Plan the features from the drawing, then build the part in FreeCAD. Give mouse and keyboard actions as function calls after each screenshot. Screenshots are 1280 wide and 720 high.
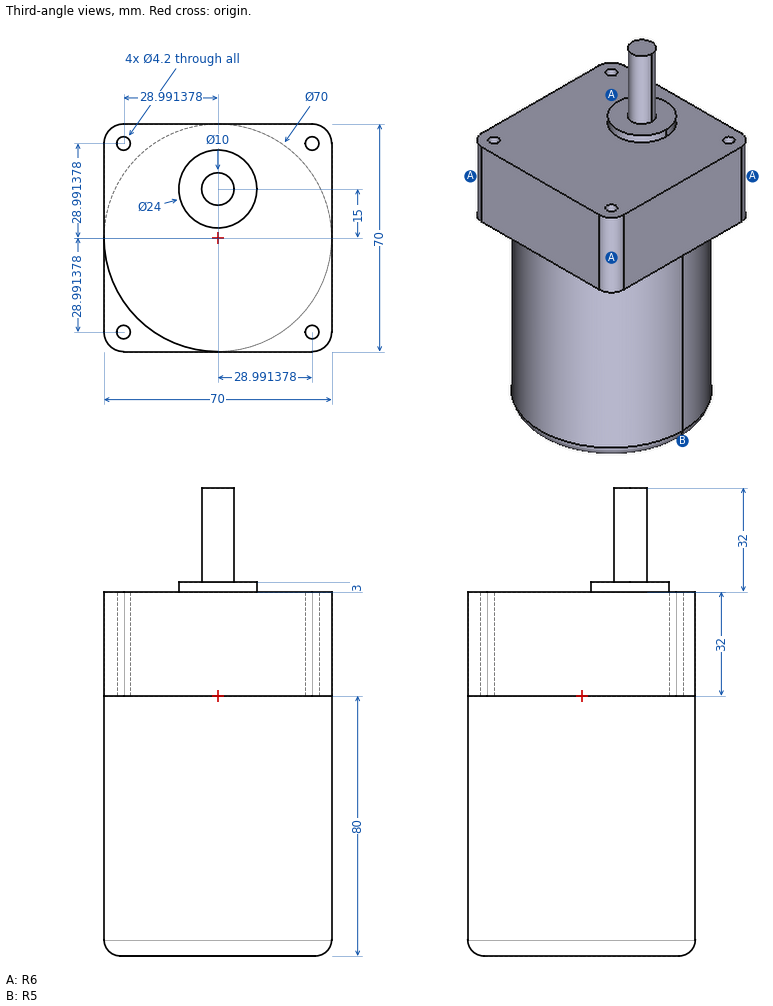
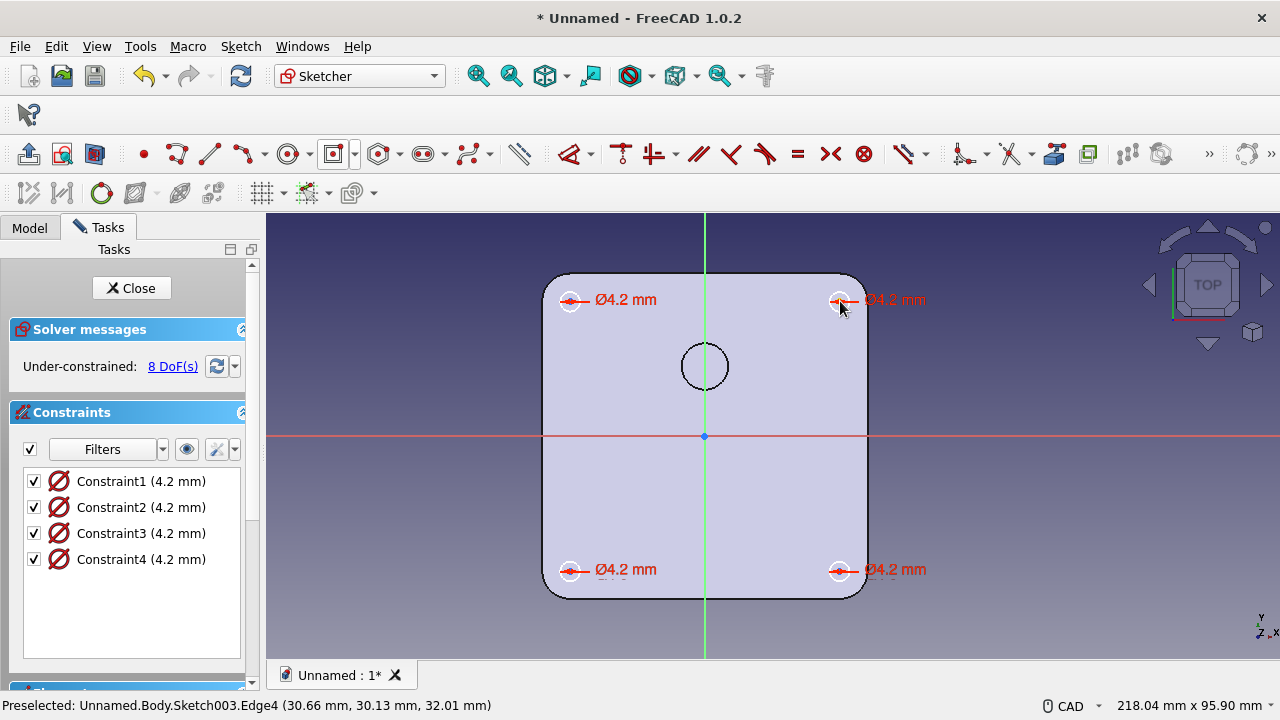
click(570, 302)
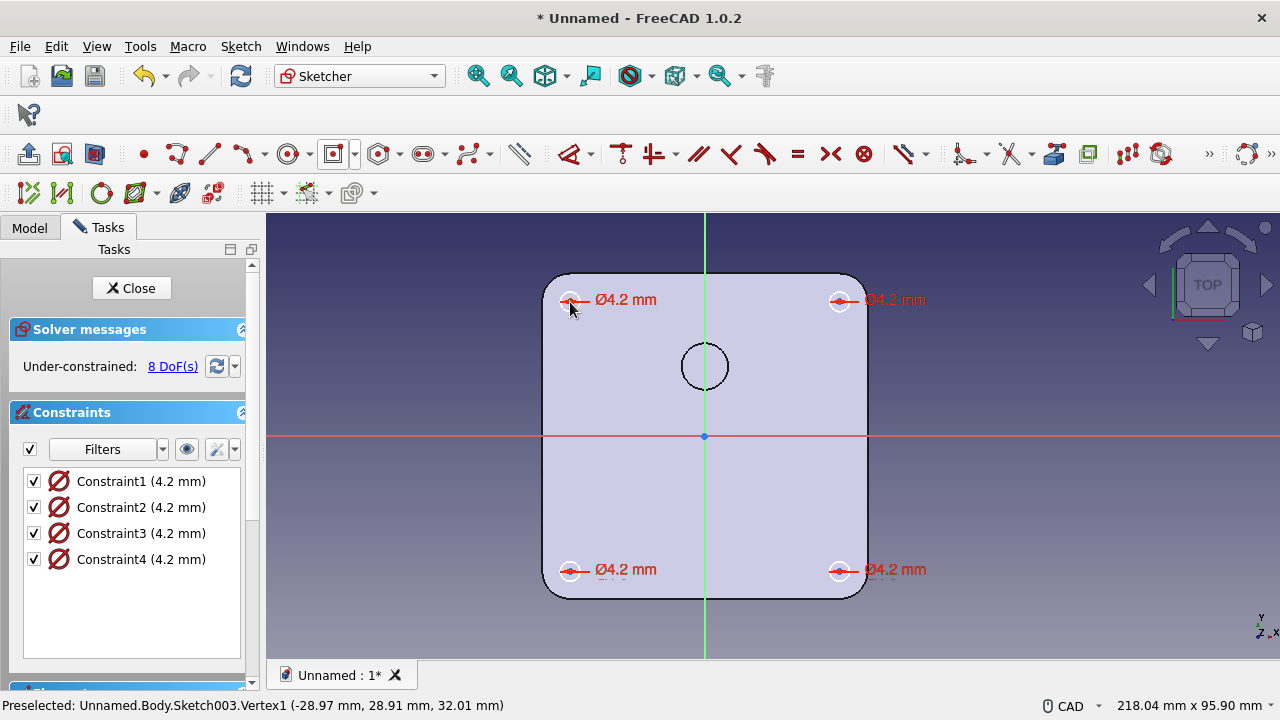
click(570, 572)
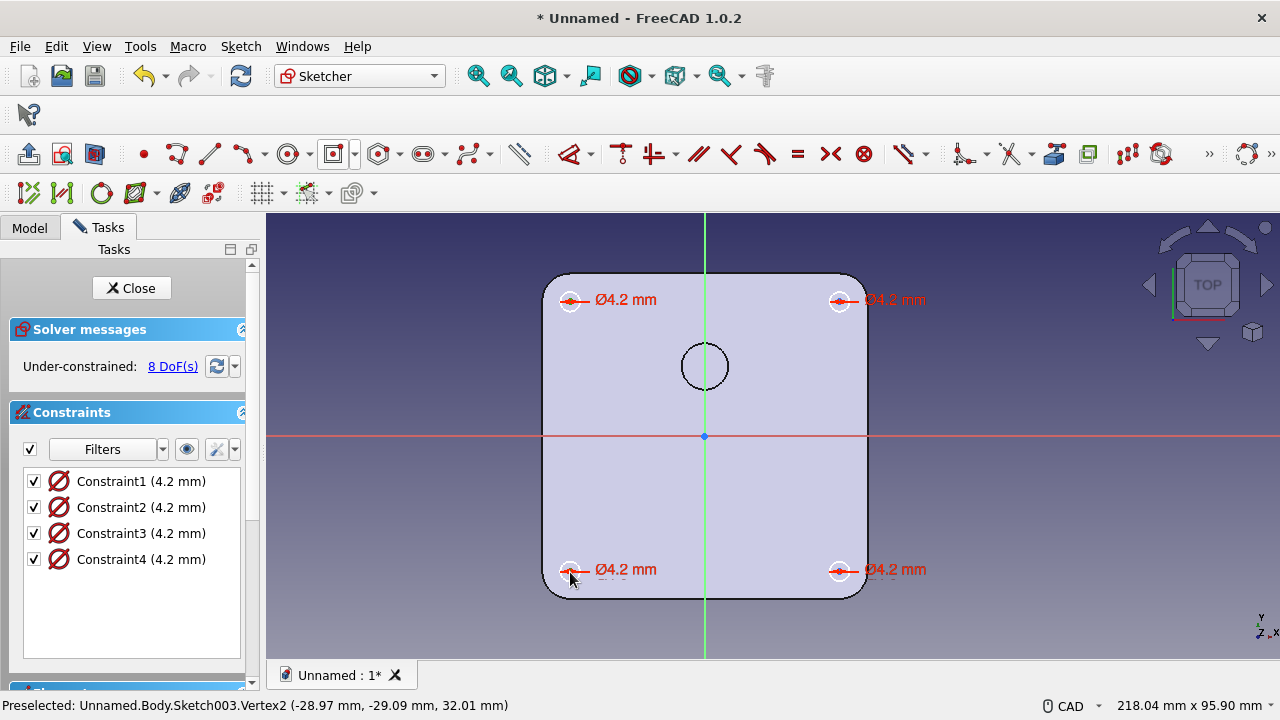
key(v)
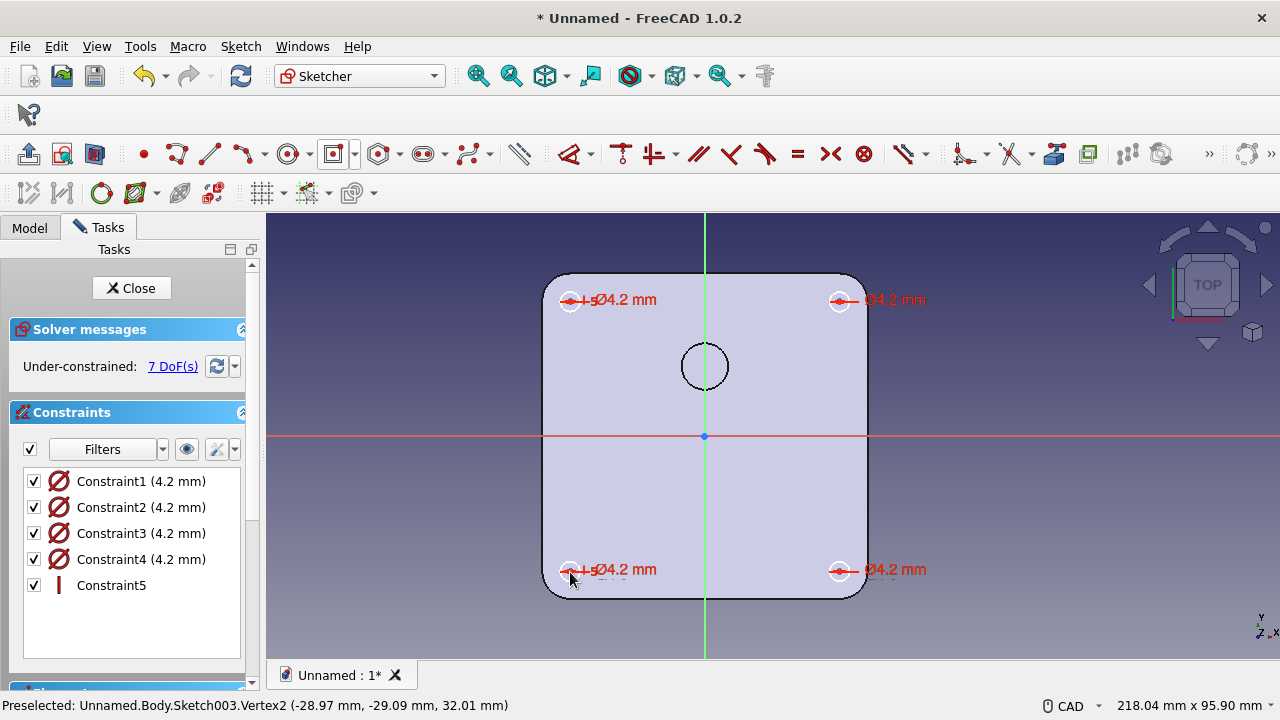
click(570, 572)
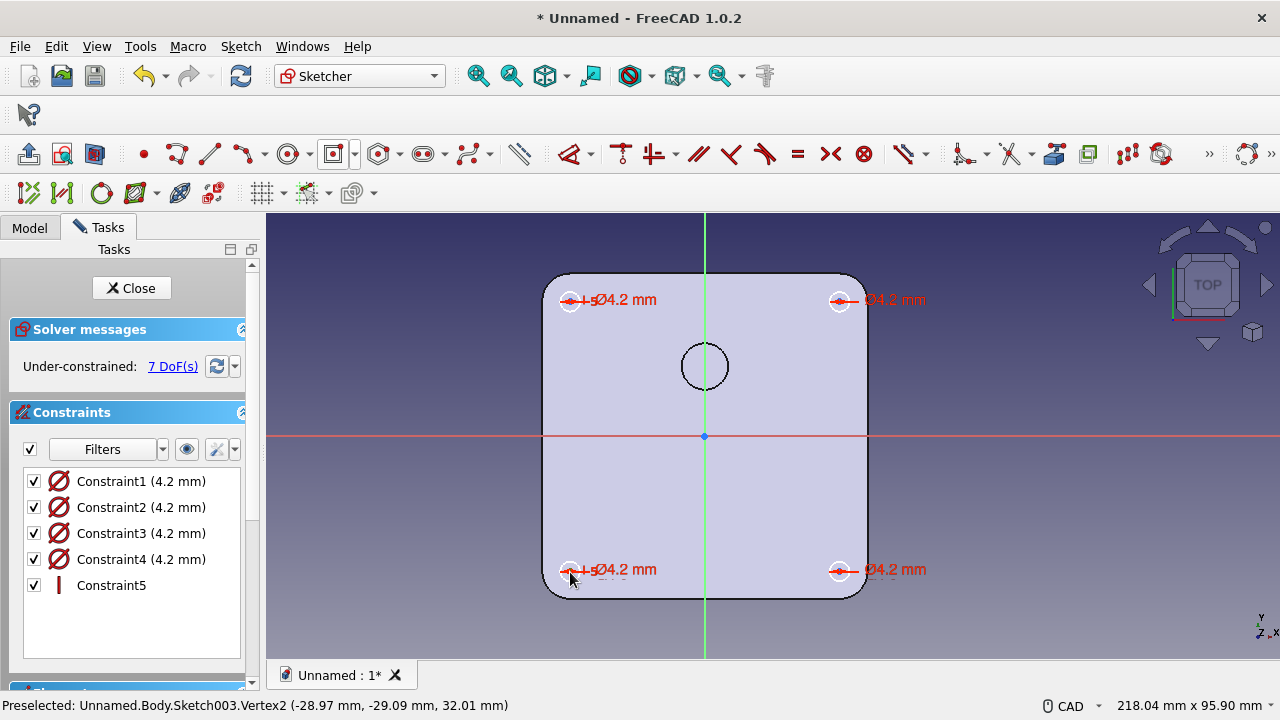
click(840, 572)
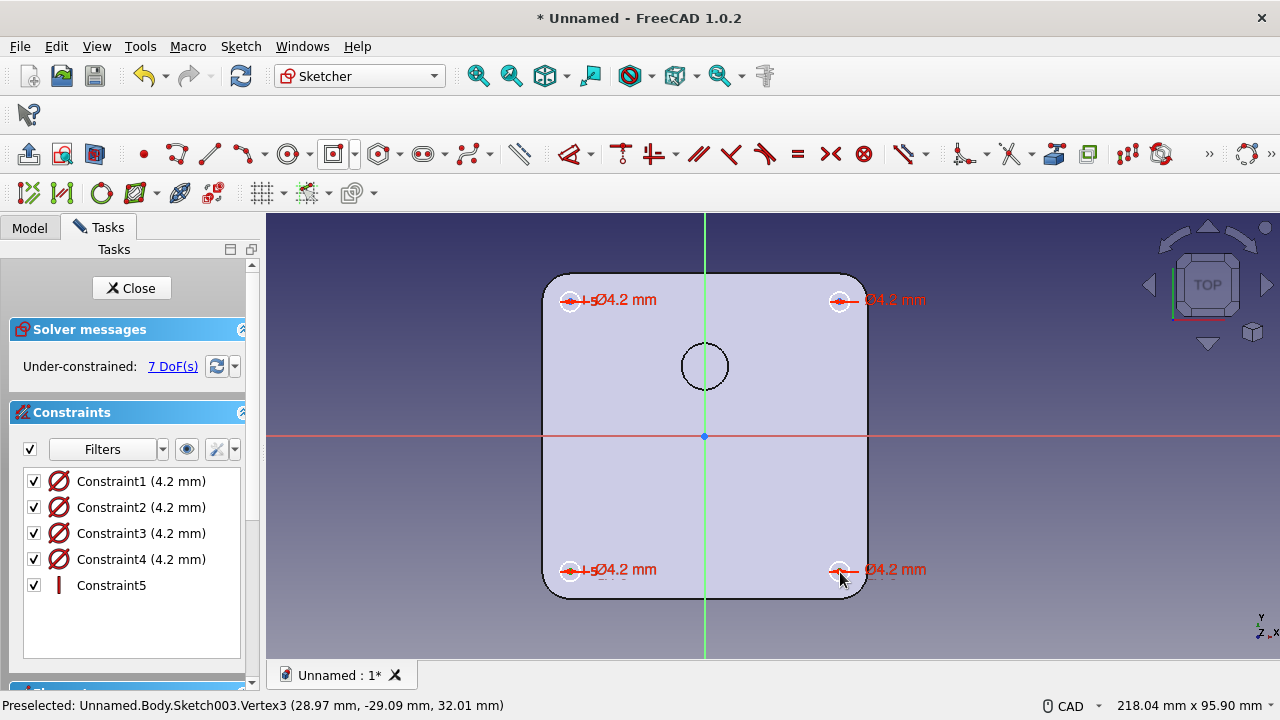
key(h)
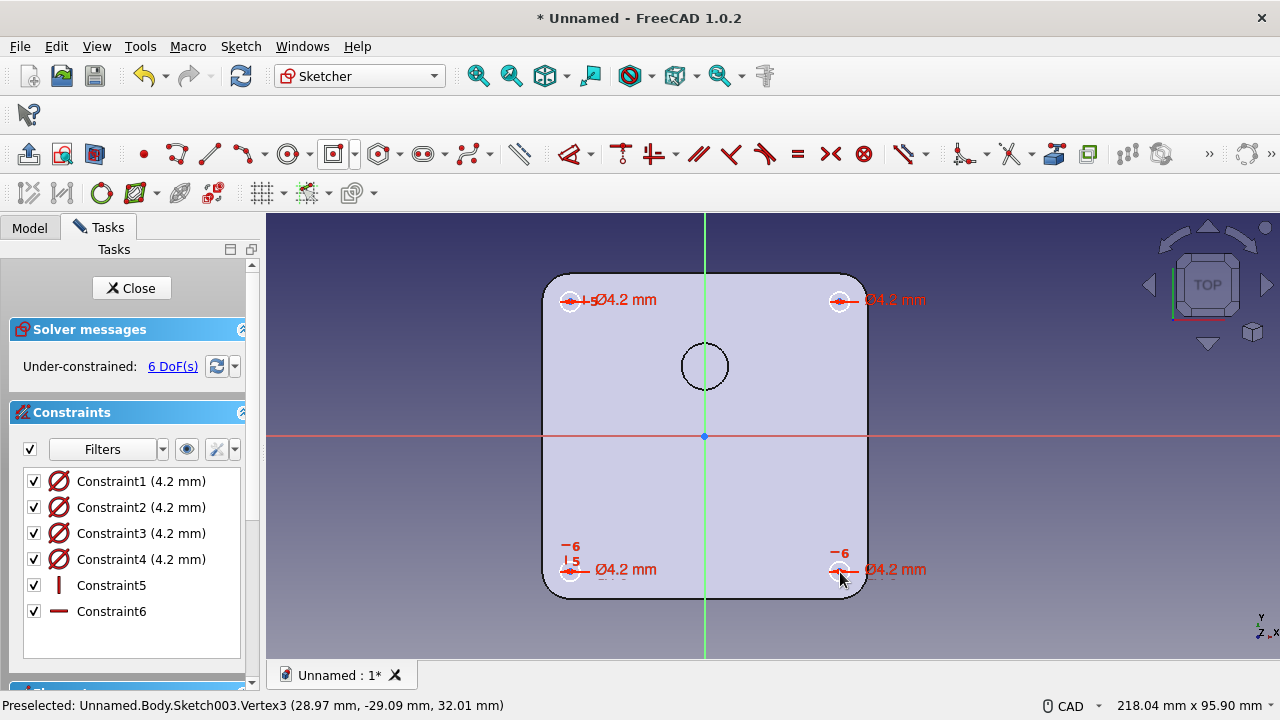
click(840, 572)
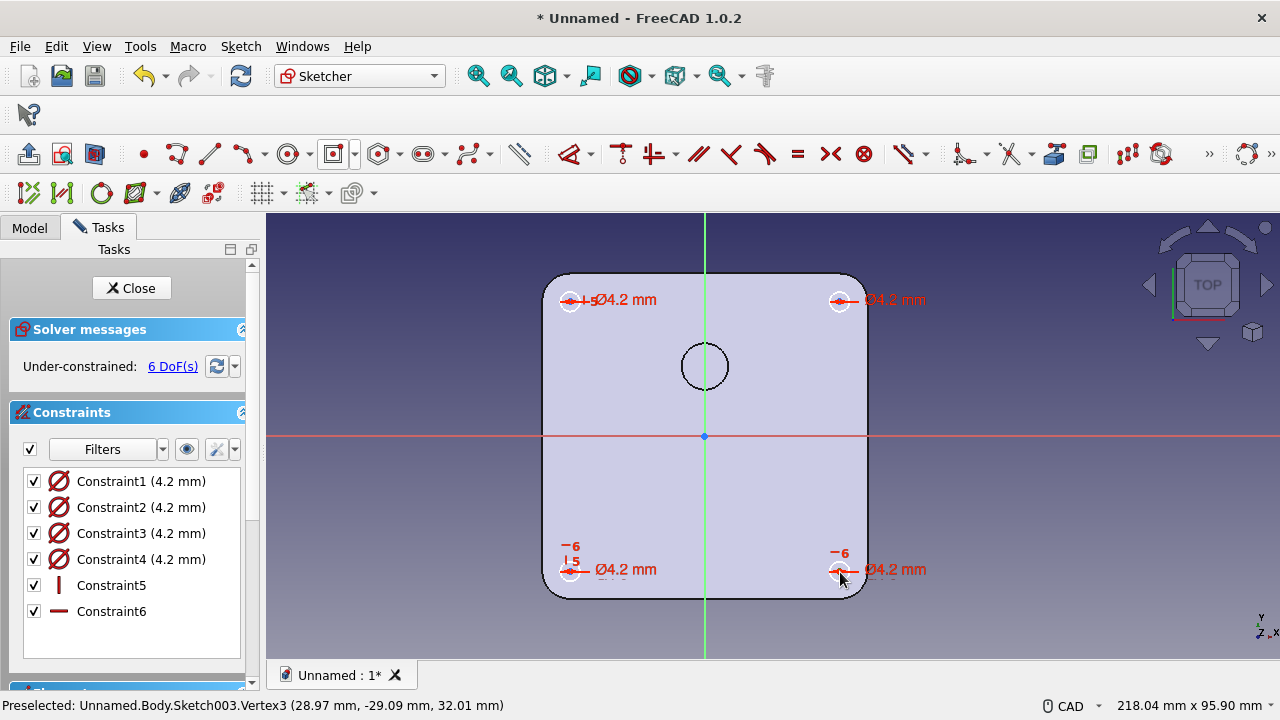
click(840, 302)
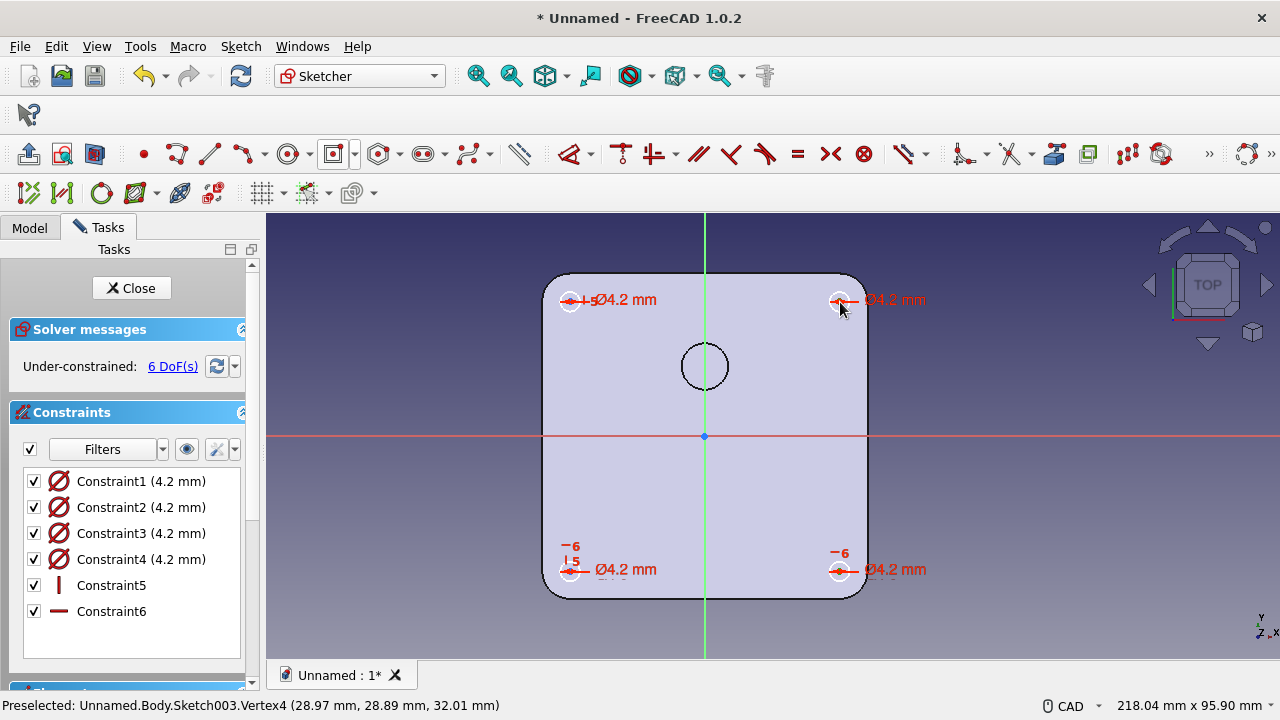
key(v)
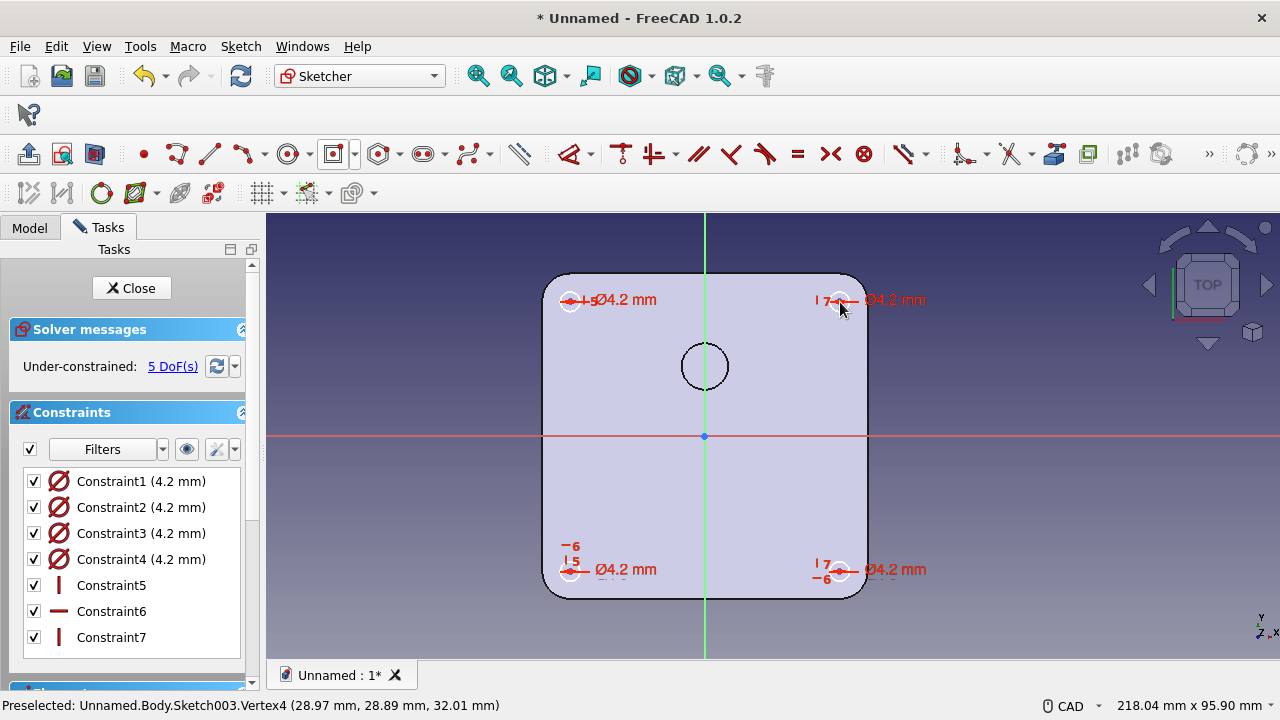
click(570, 302)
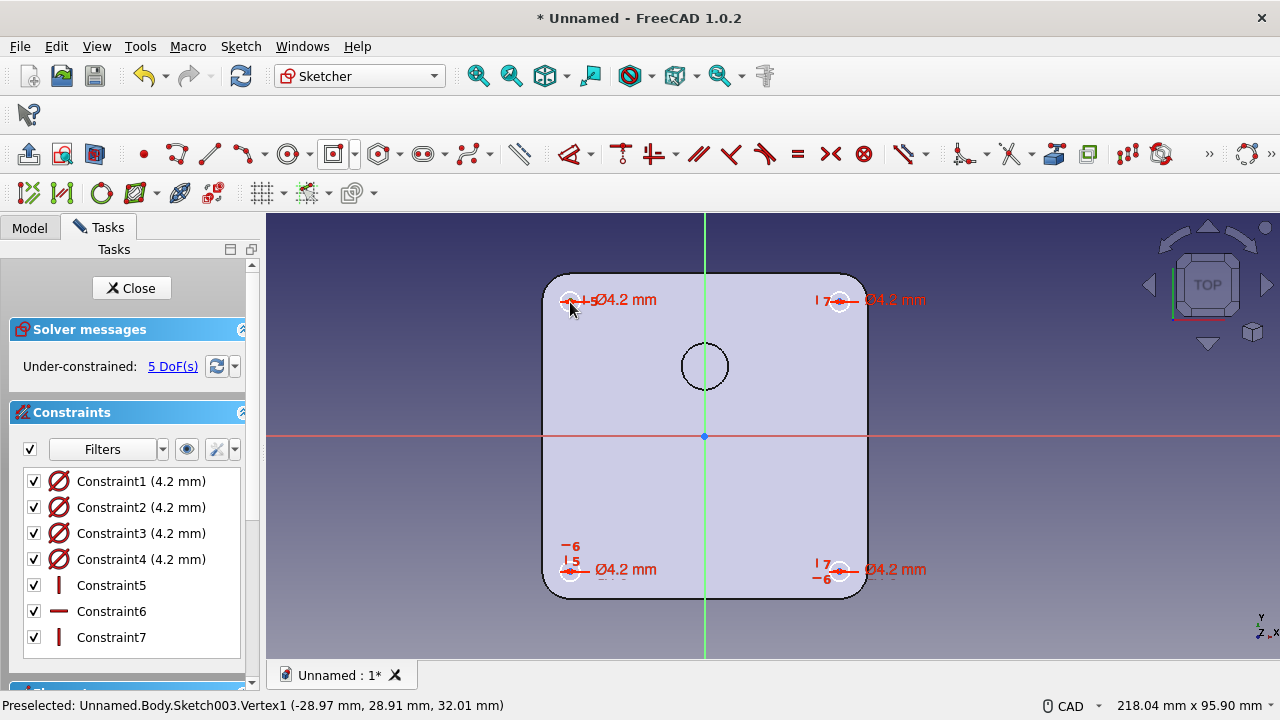
click(840, 302)